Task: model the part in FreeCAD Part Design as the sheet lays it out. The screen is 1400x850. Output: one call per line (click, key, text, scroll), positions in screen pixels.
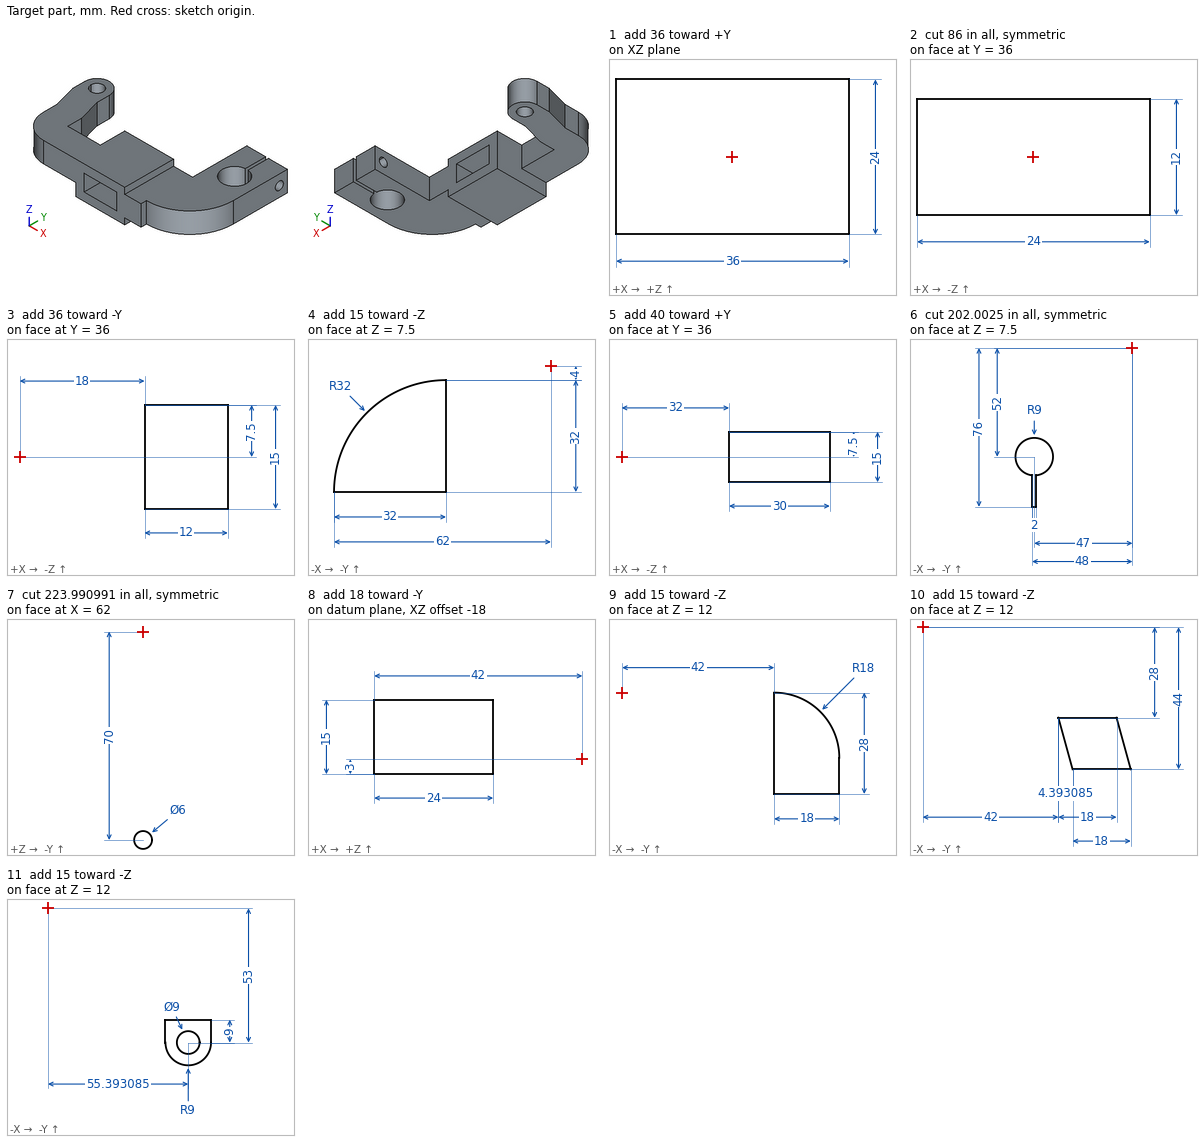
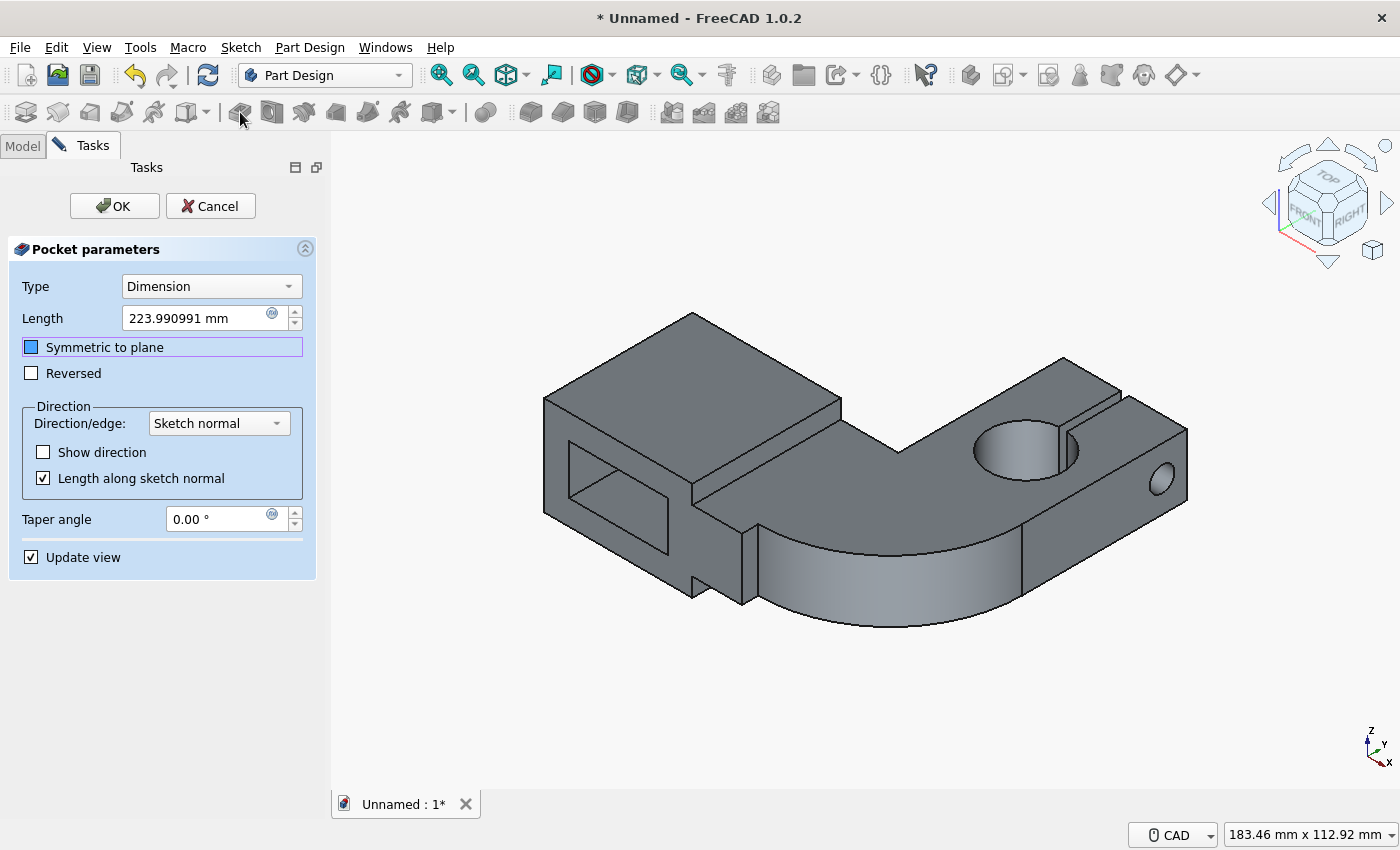
click(30, 347)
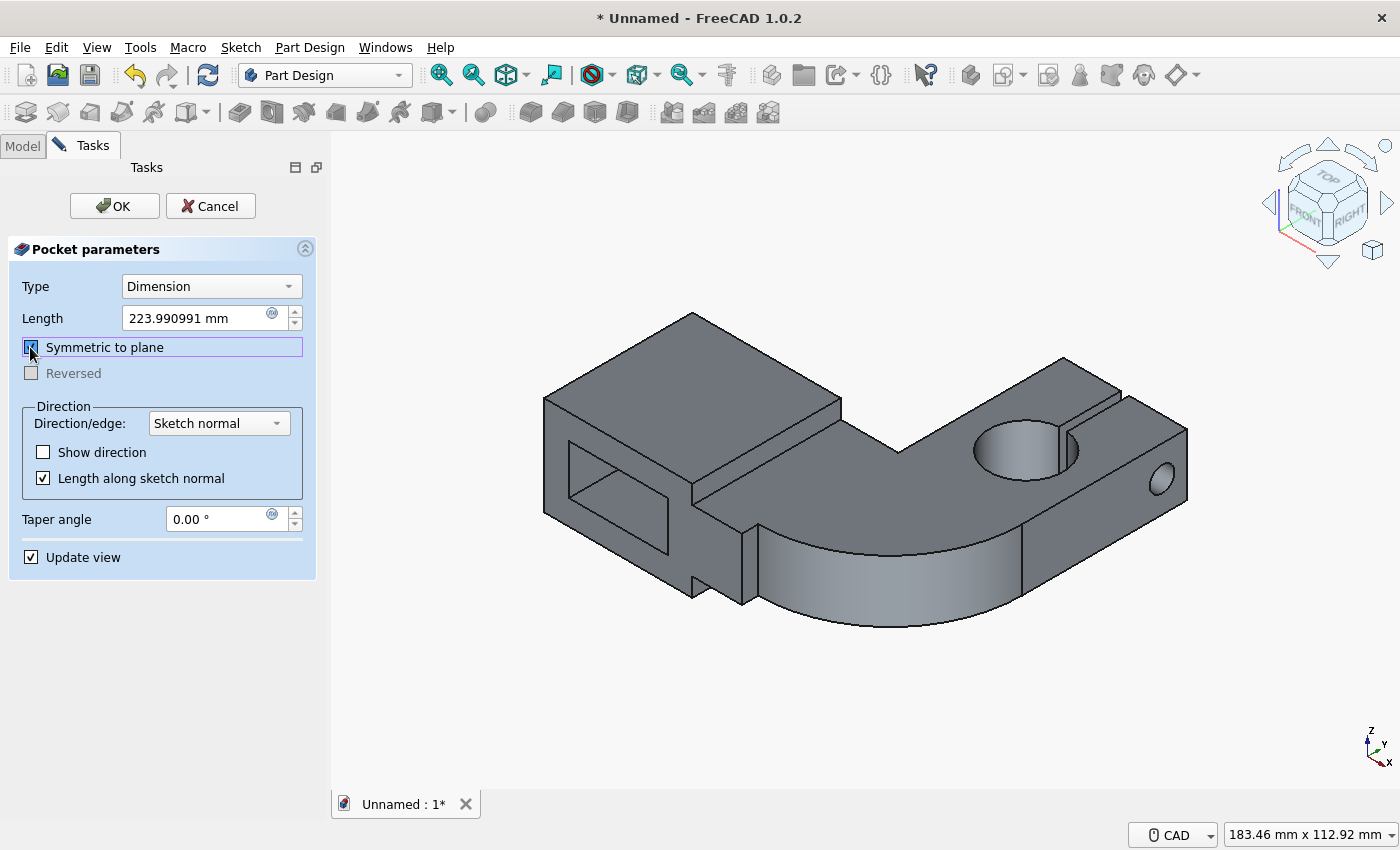
click(115, 206)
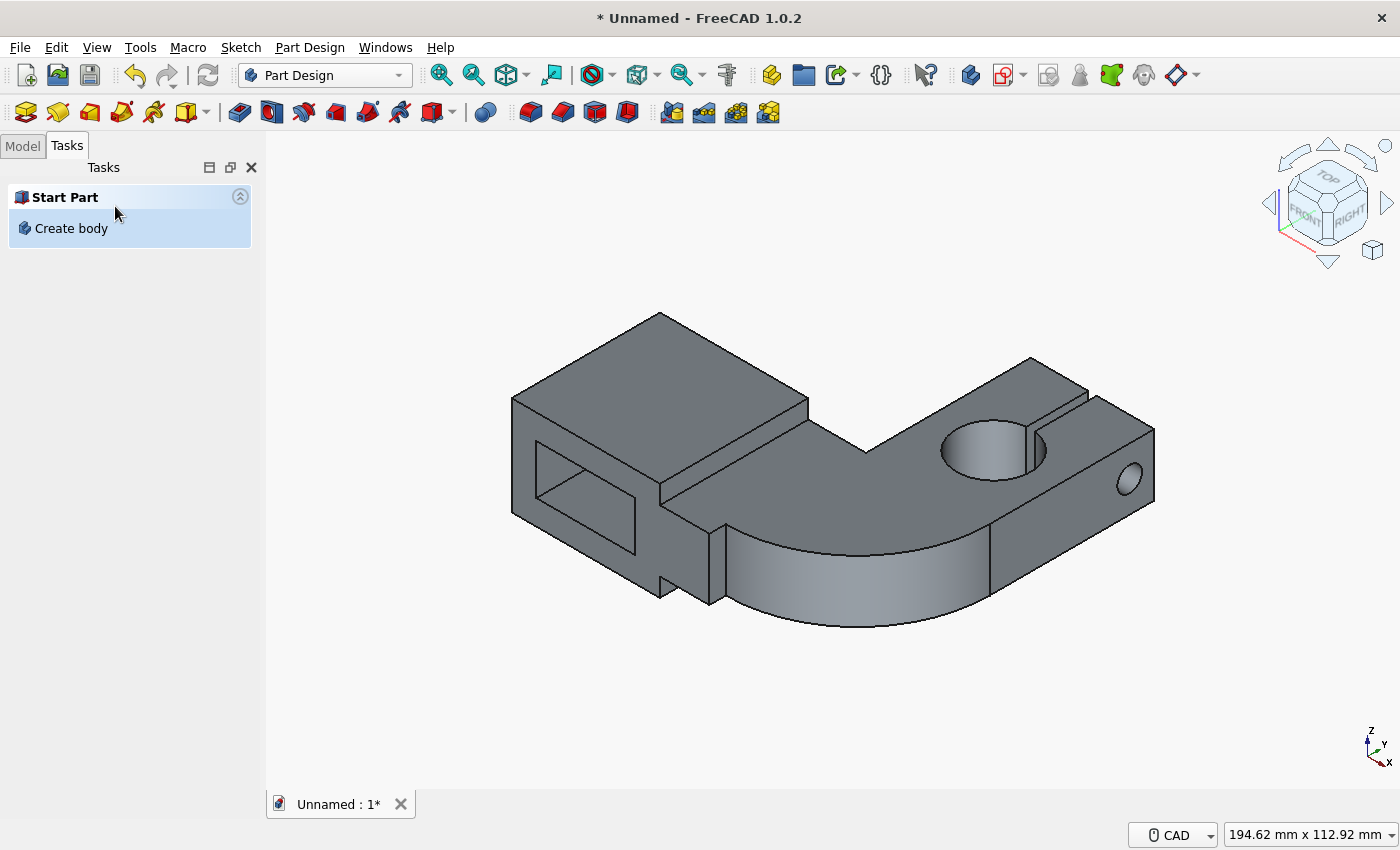
click(23, 145)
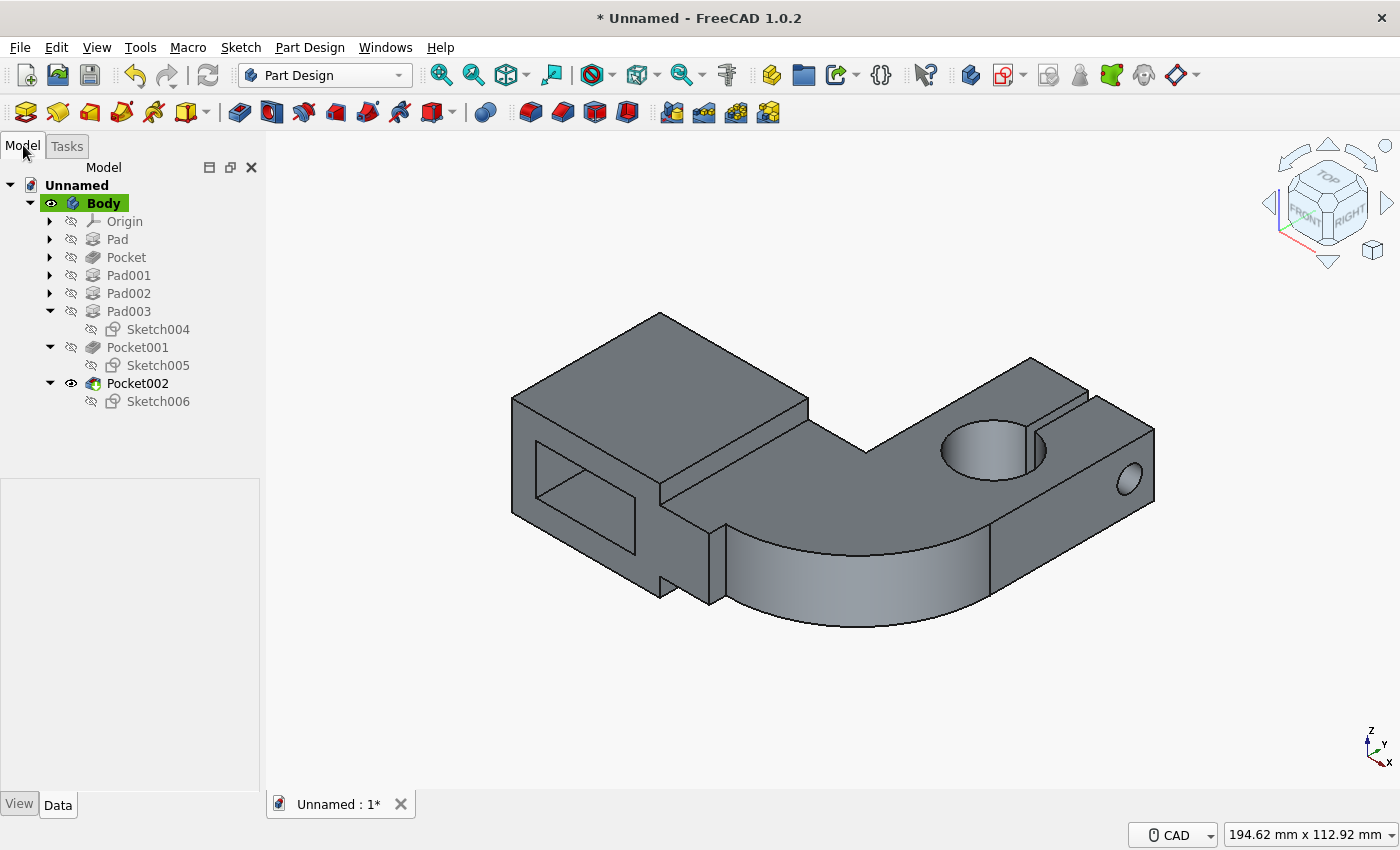
click(50, 221)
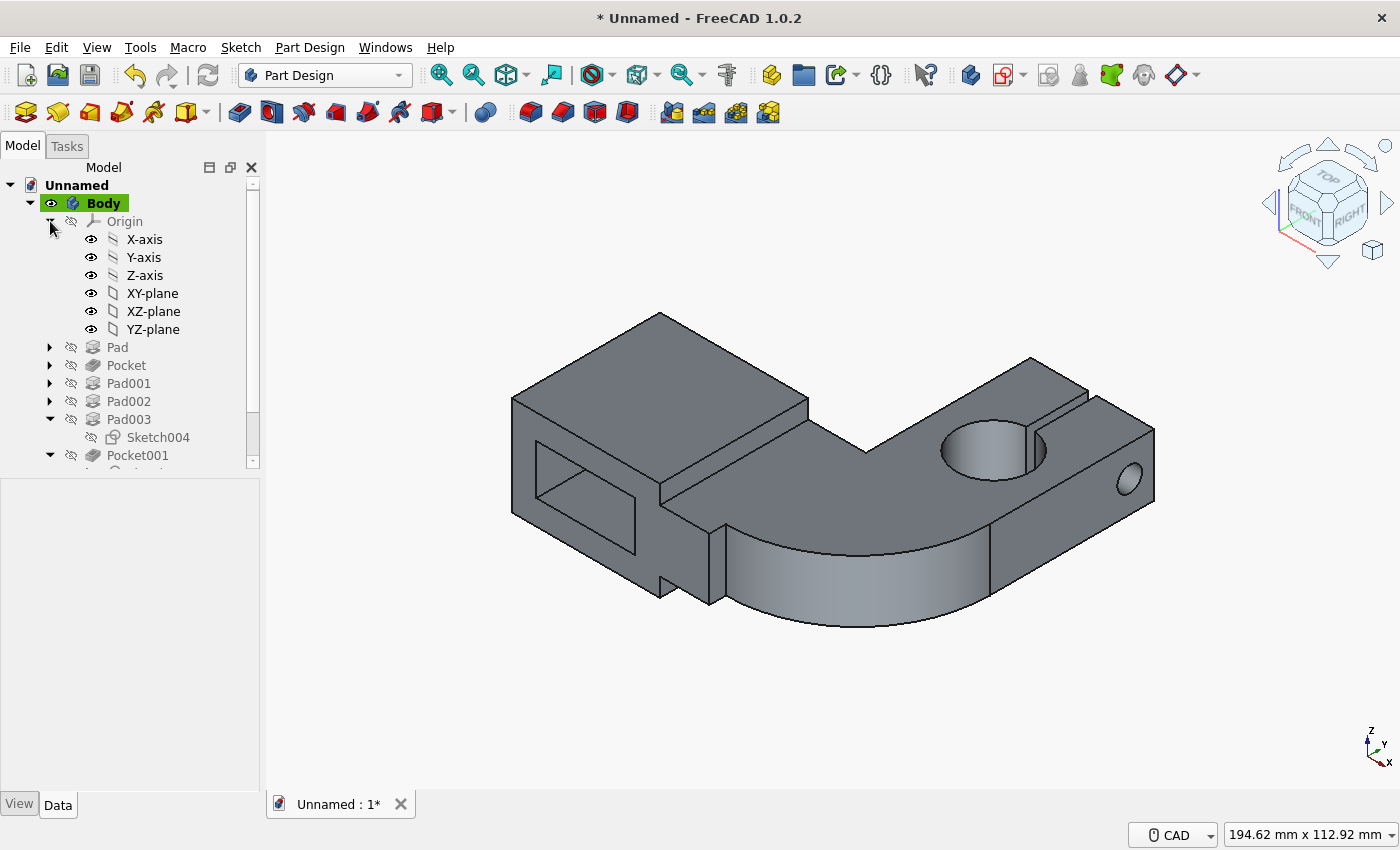
click(136, 311)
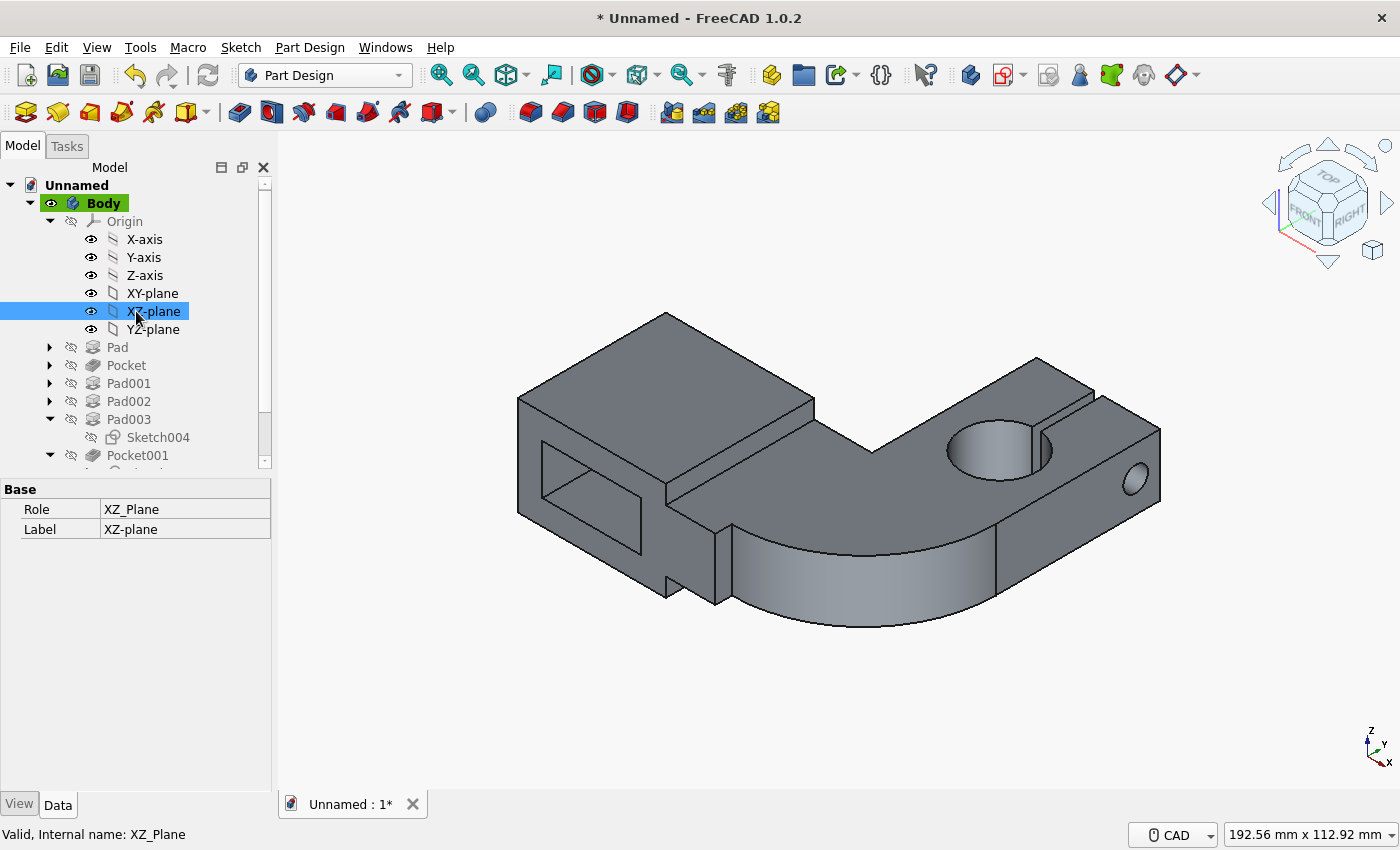
click(1176, 76)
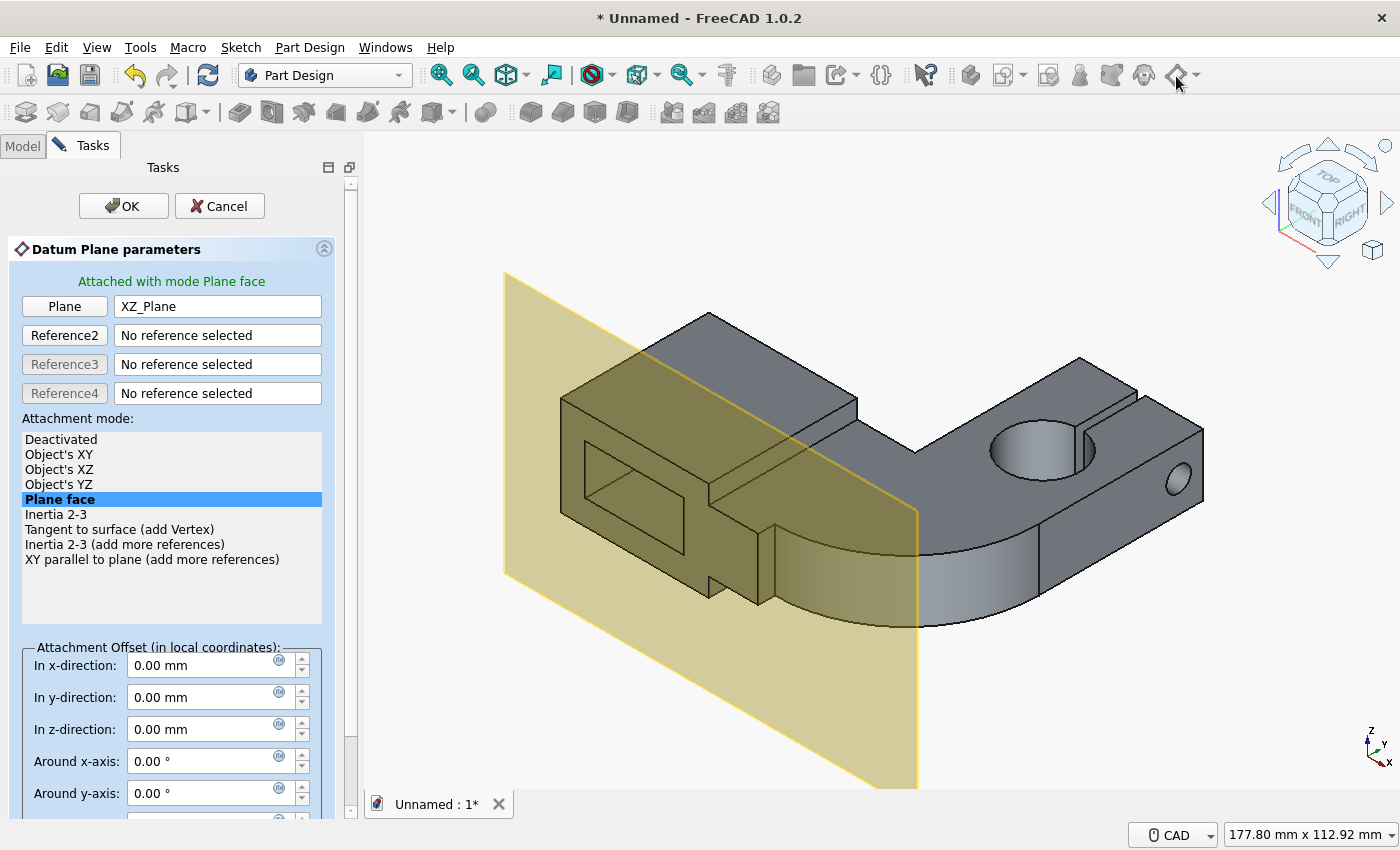
triple_click(210, 729)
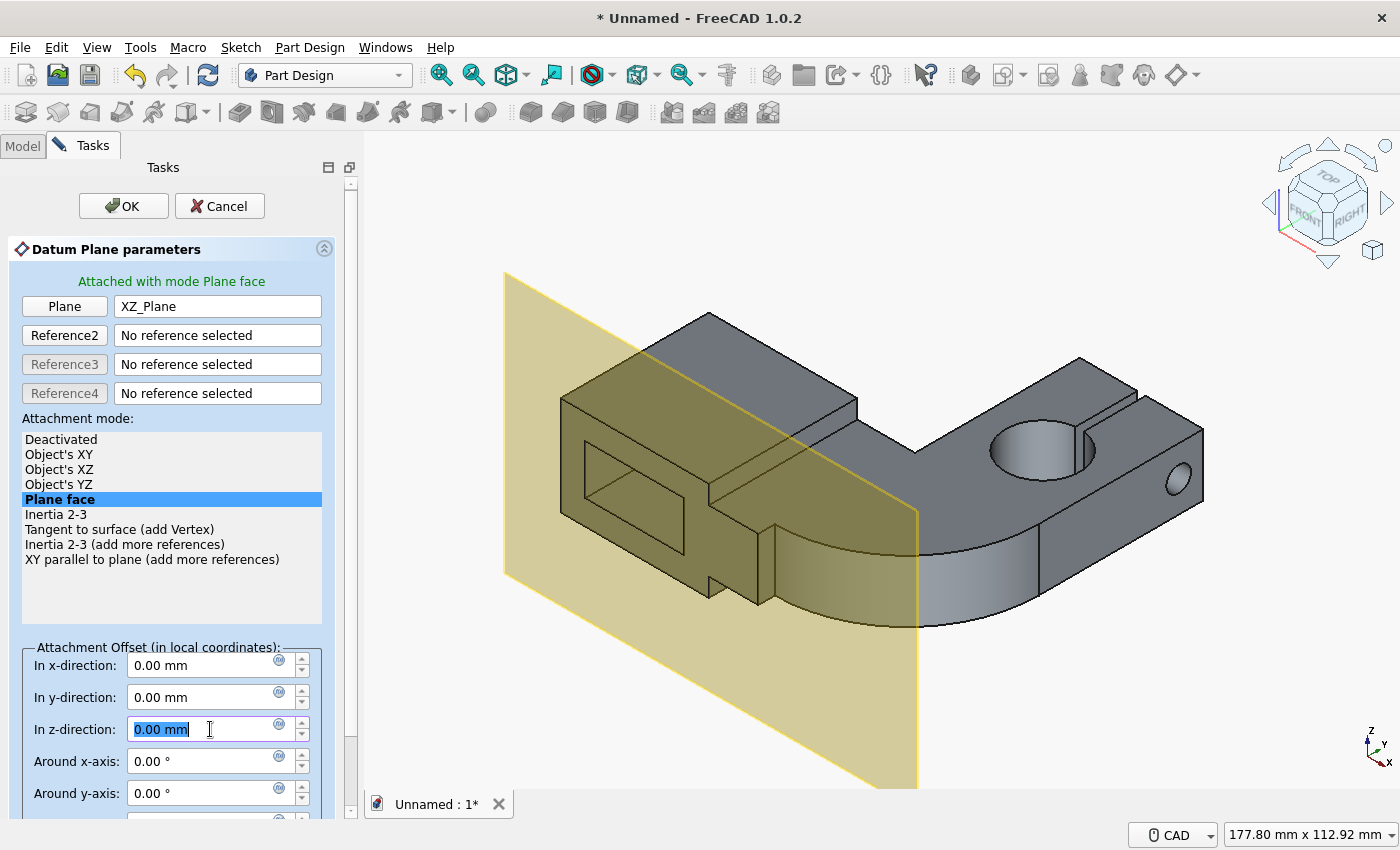
text(-18)
key(Tab)